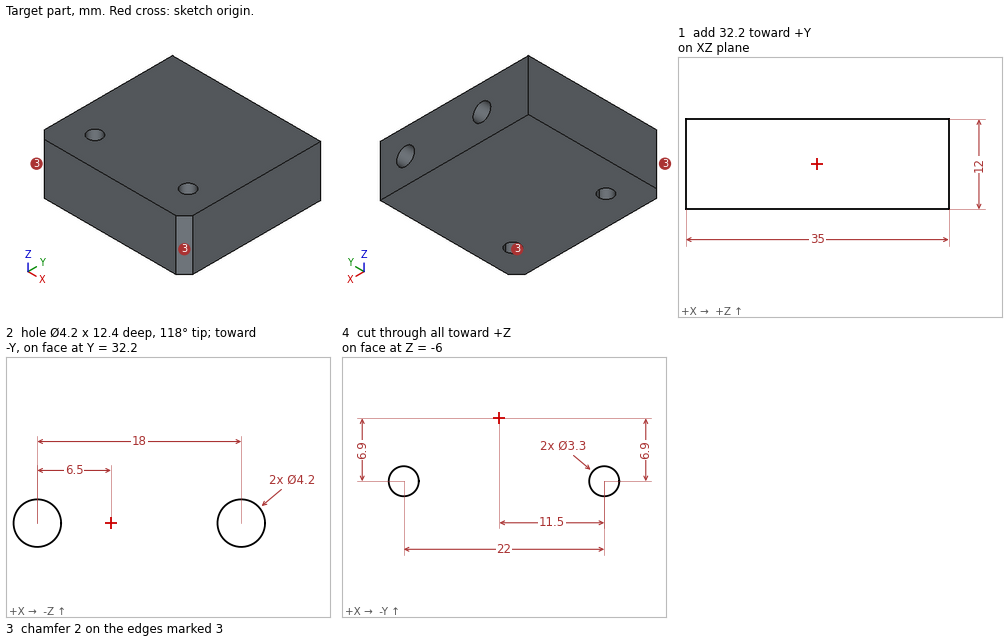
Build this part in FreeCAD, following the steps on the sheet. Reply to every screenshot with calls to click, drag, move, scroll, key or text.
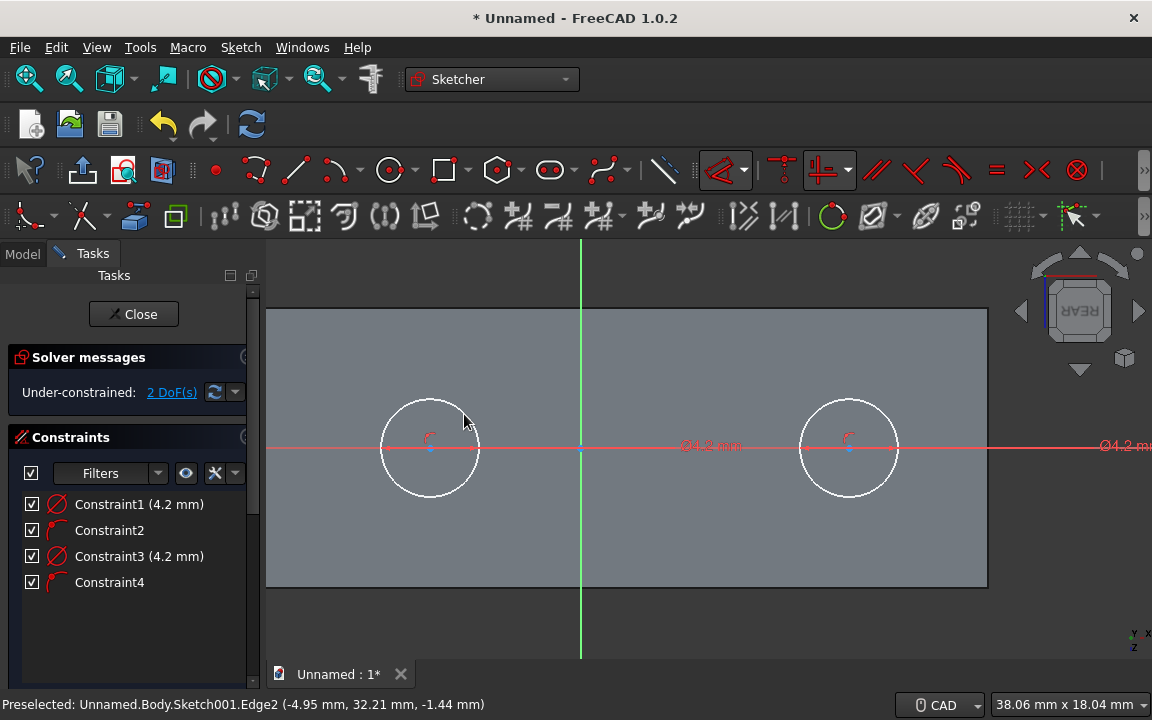
key(d)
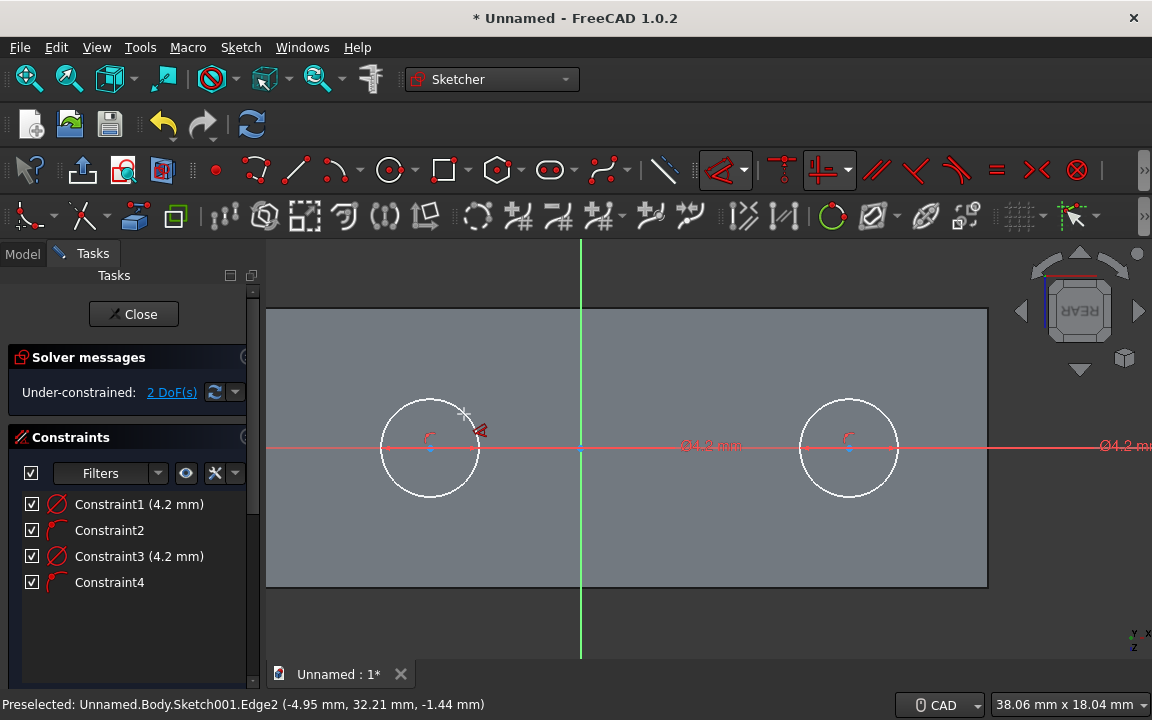
click(430, 448)
click(505, 482)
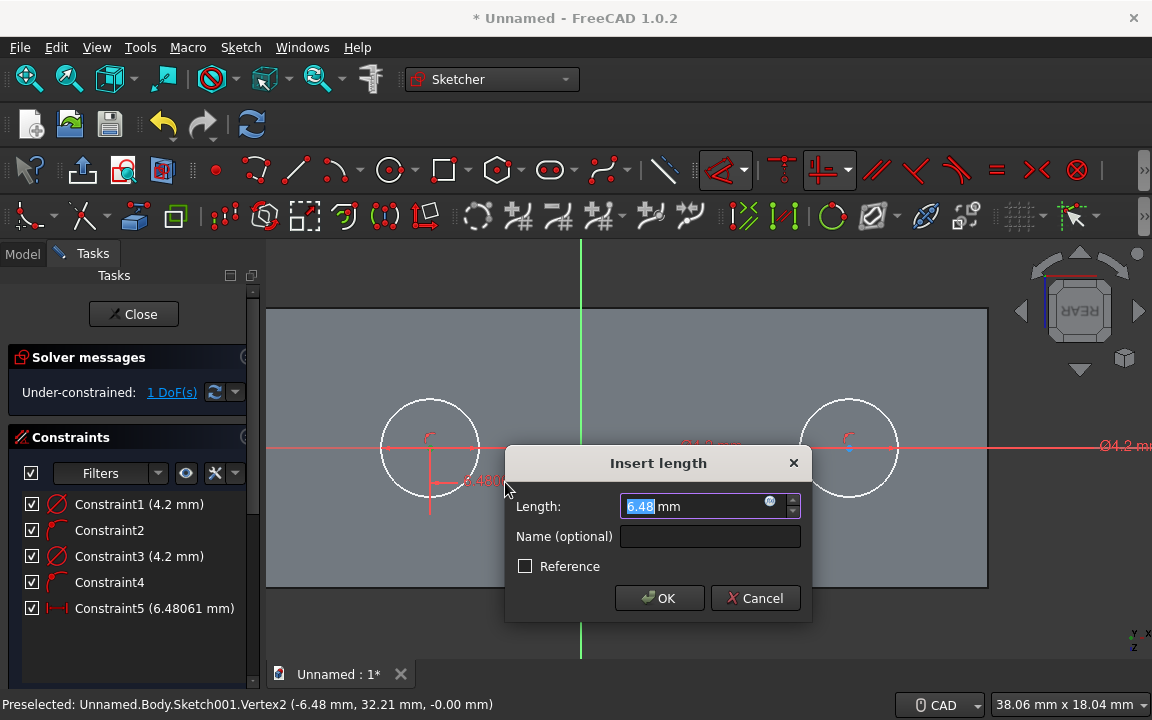
text(6.5)
key(Return)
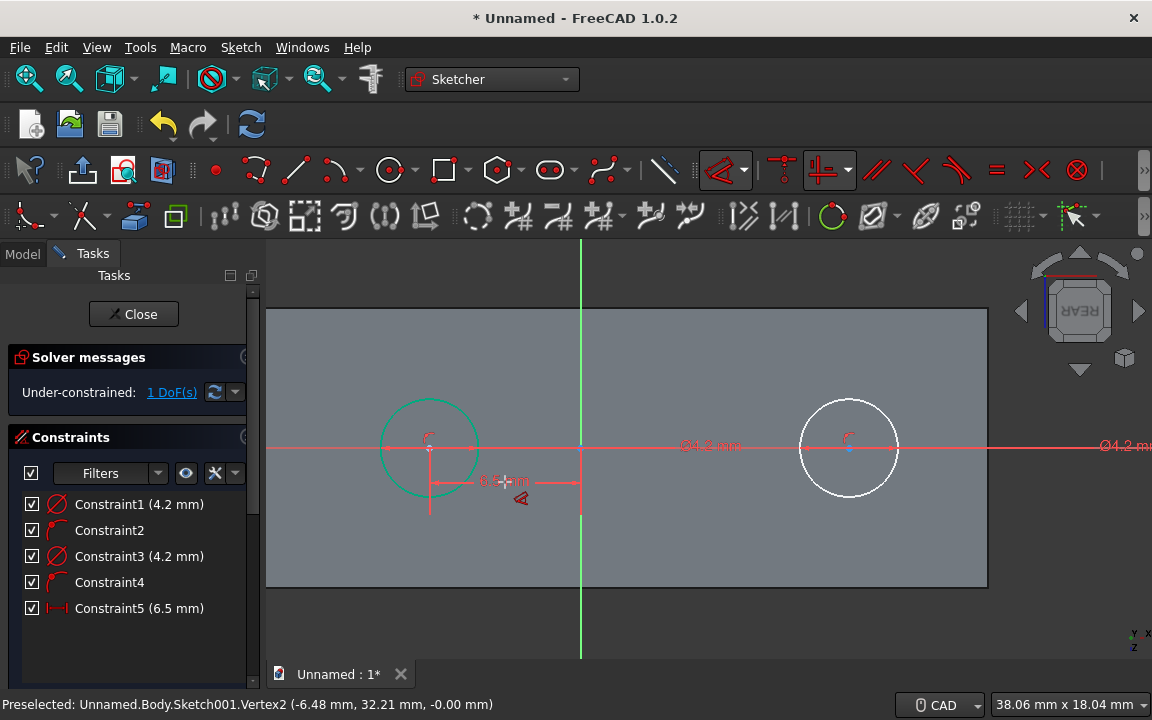
click(849, 448)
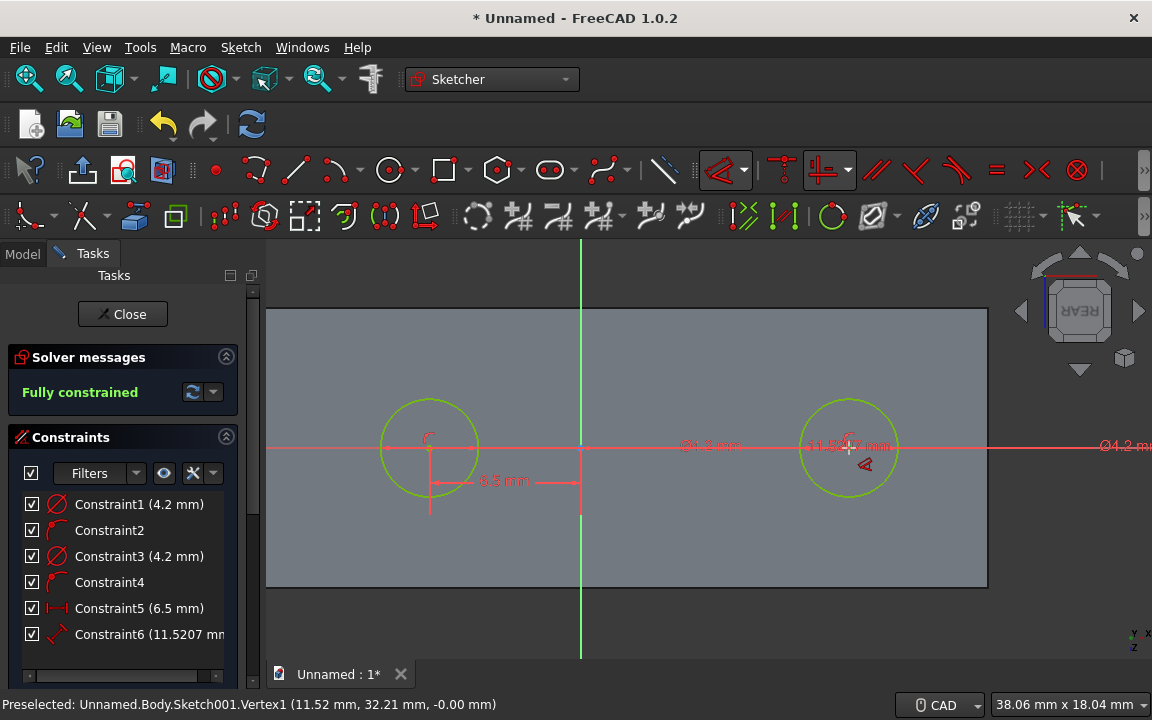
click(430, 448)
click(639, 482)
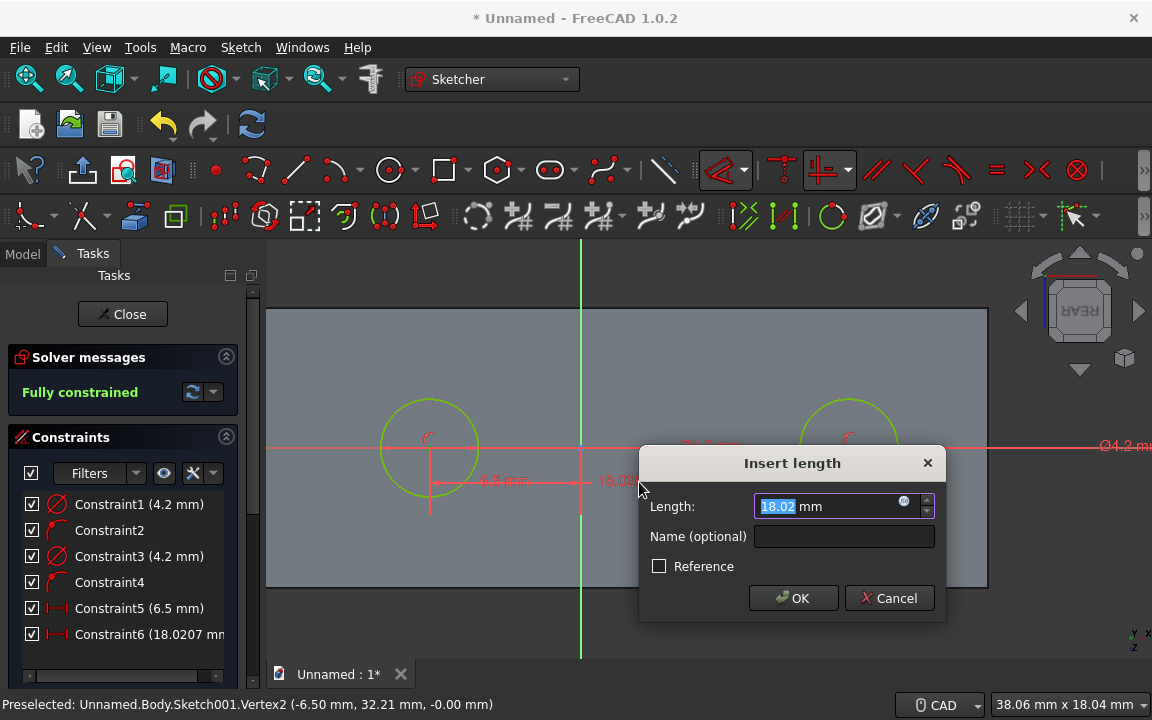
text(18)
key(Return)
key(Escape)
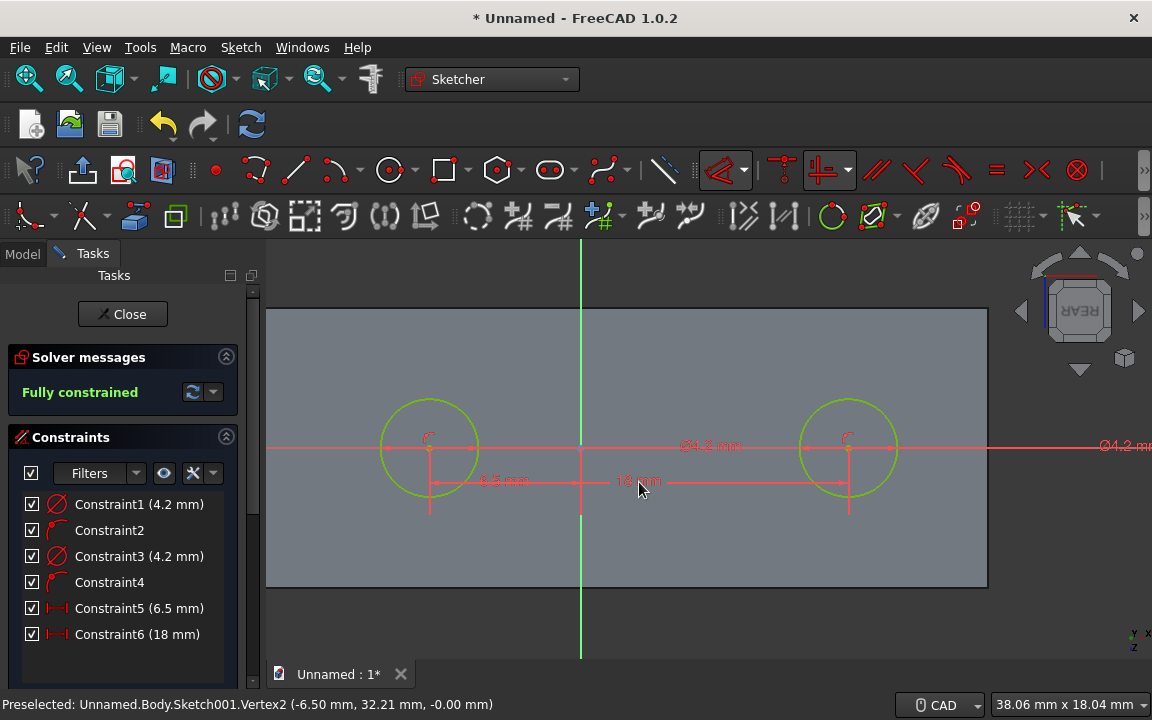
click(123, 314)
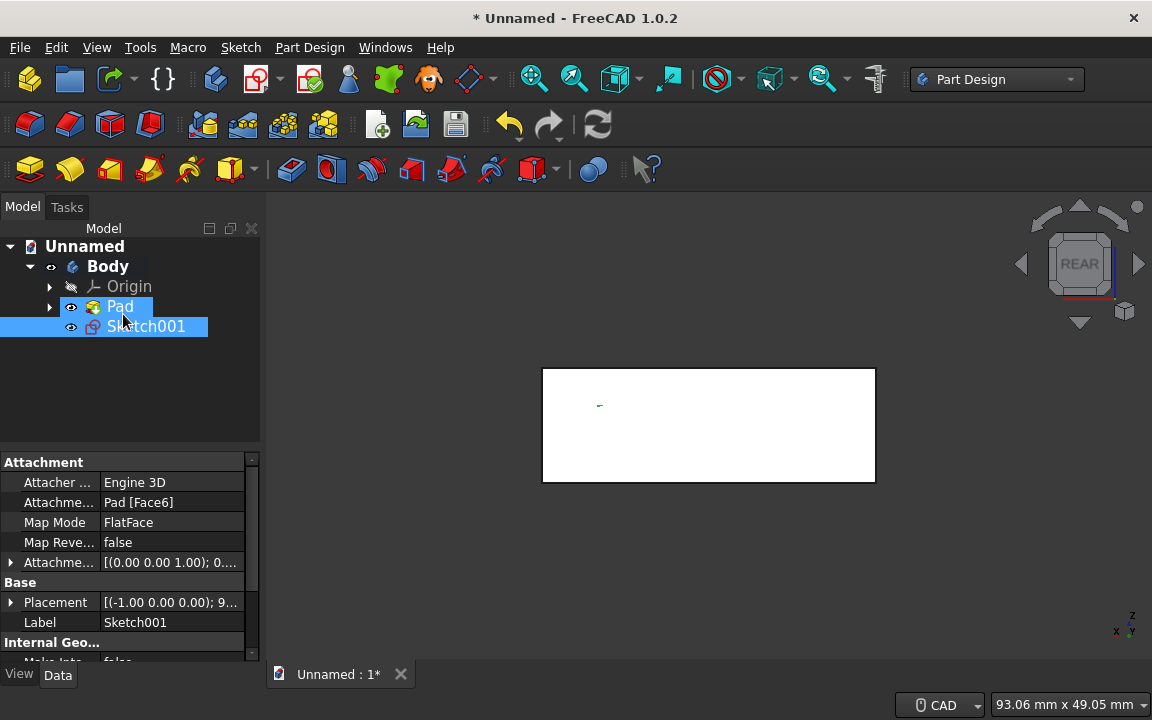
click(332, 170)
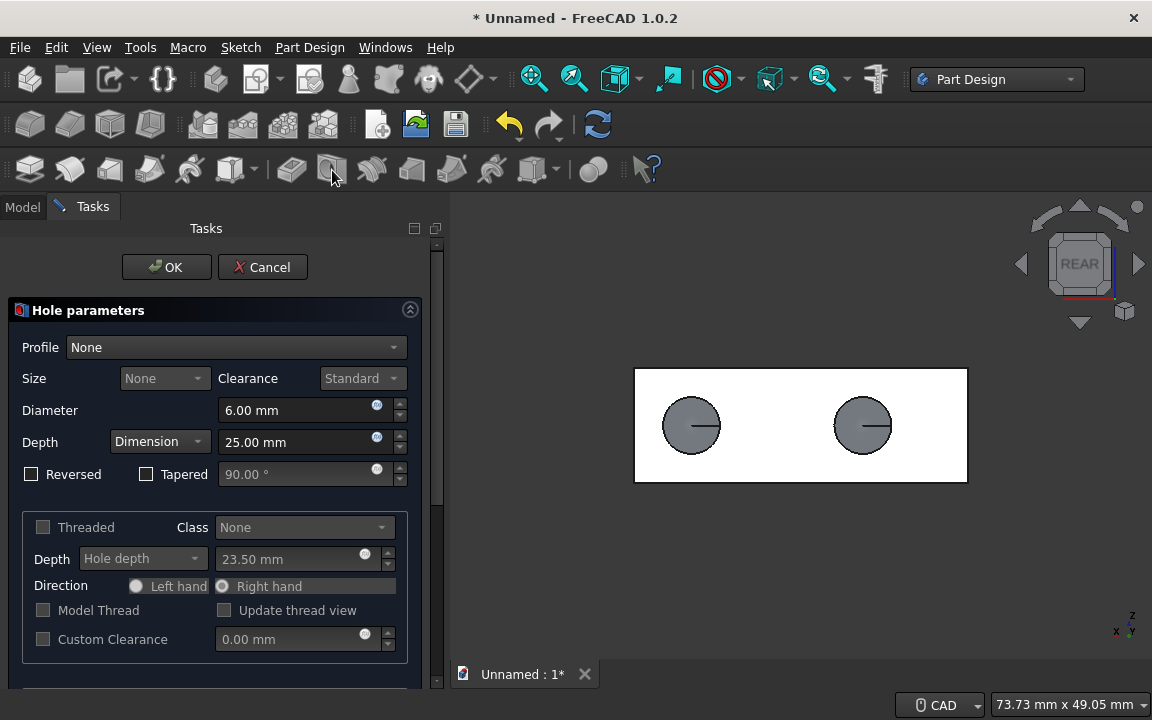
triple_click(305, 410)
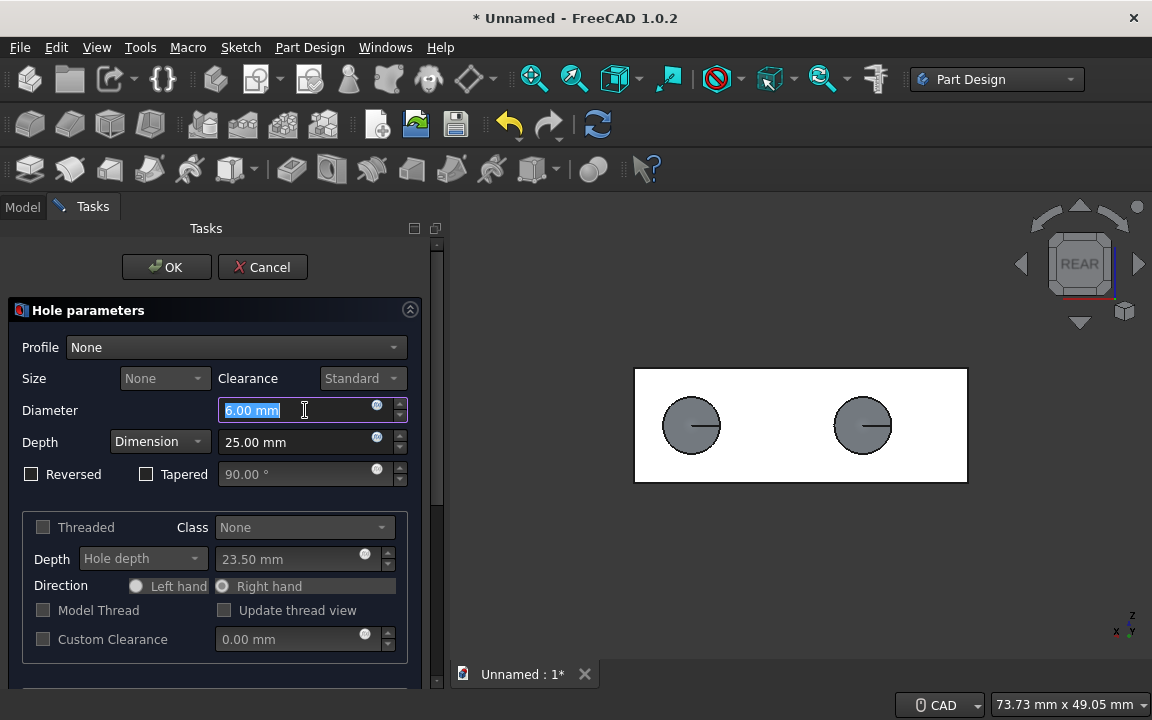
text(4.2)
key(Tab)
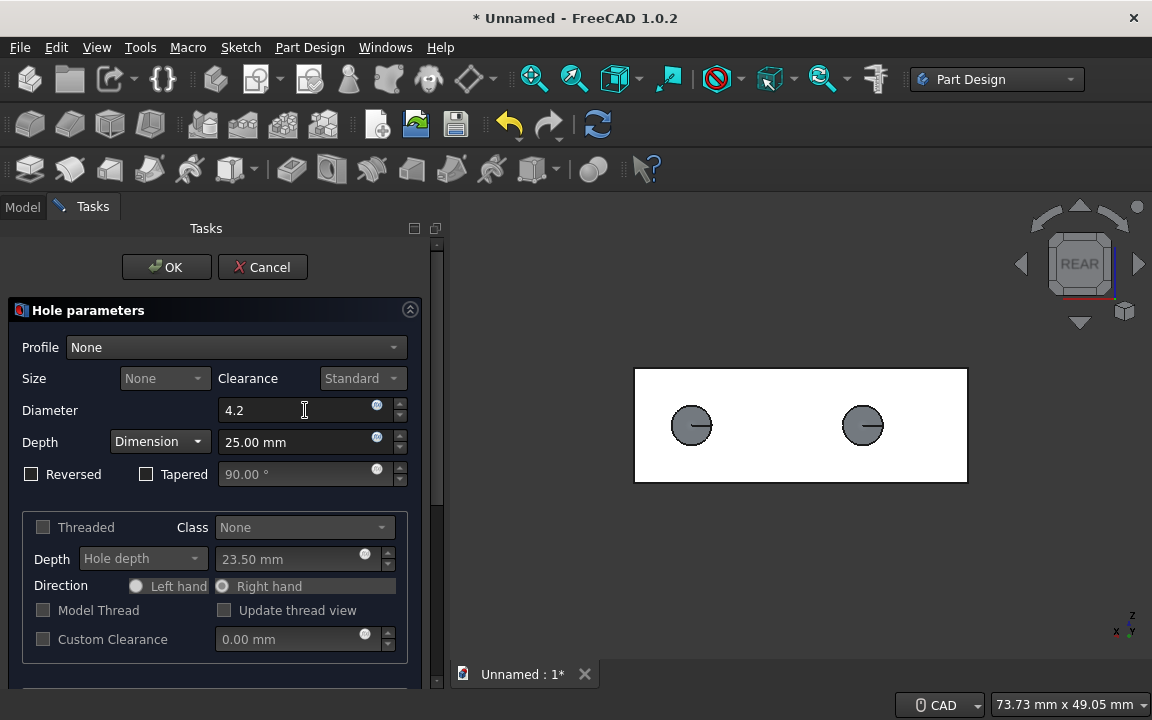
triple_click(305, 442)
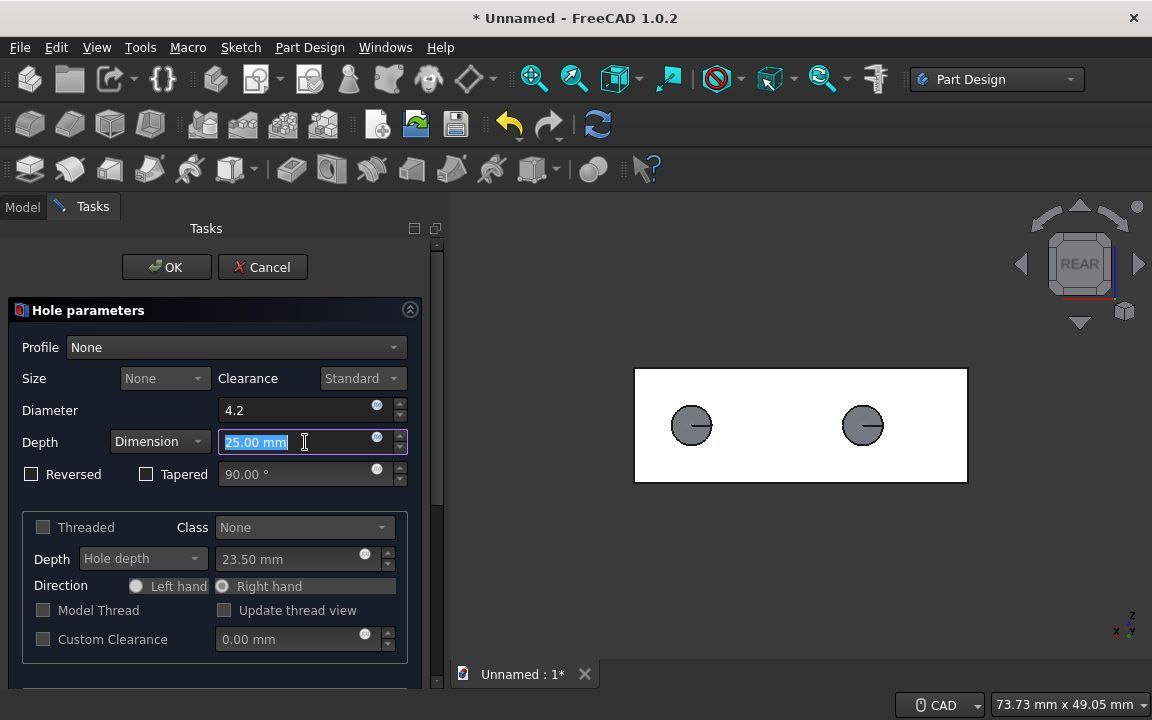
text(12.4)
key(Tab)